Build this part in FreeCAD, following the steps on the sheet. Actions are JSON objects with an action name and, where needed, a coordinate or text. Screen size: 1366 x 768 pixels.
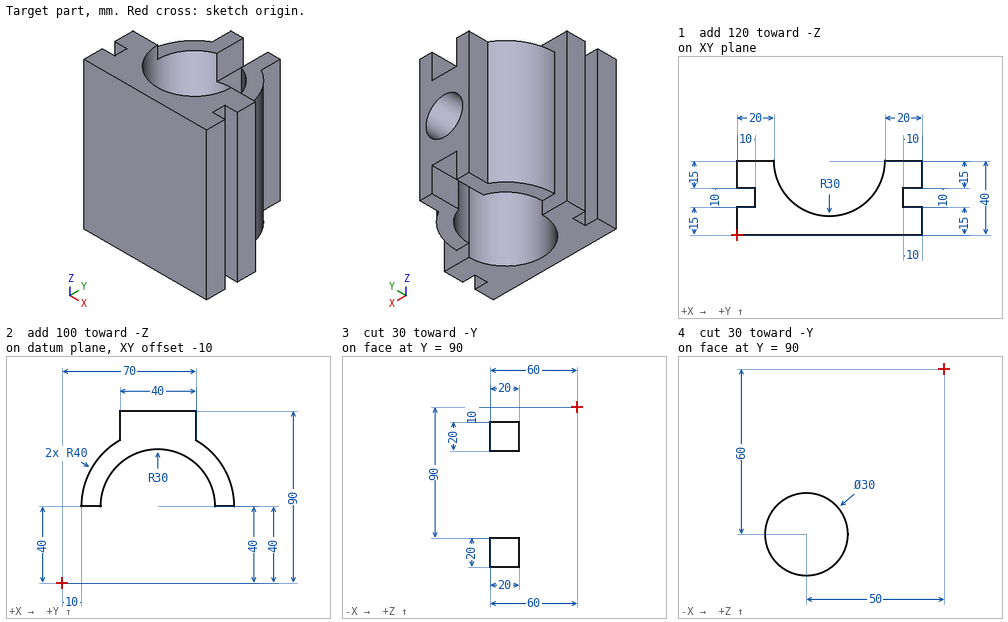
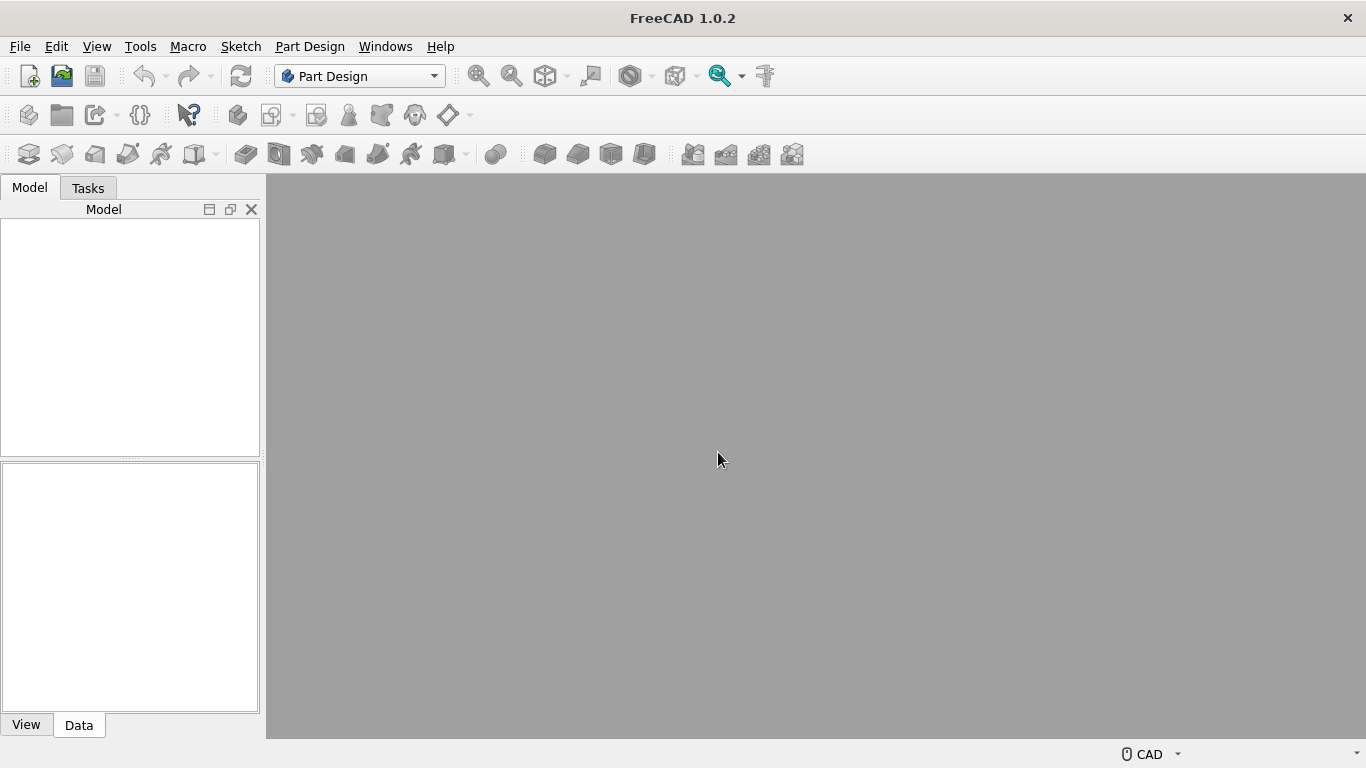
{"action": "left_click", "coordinate": [29, 76]}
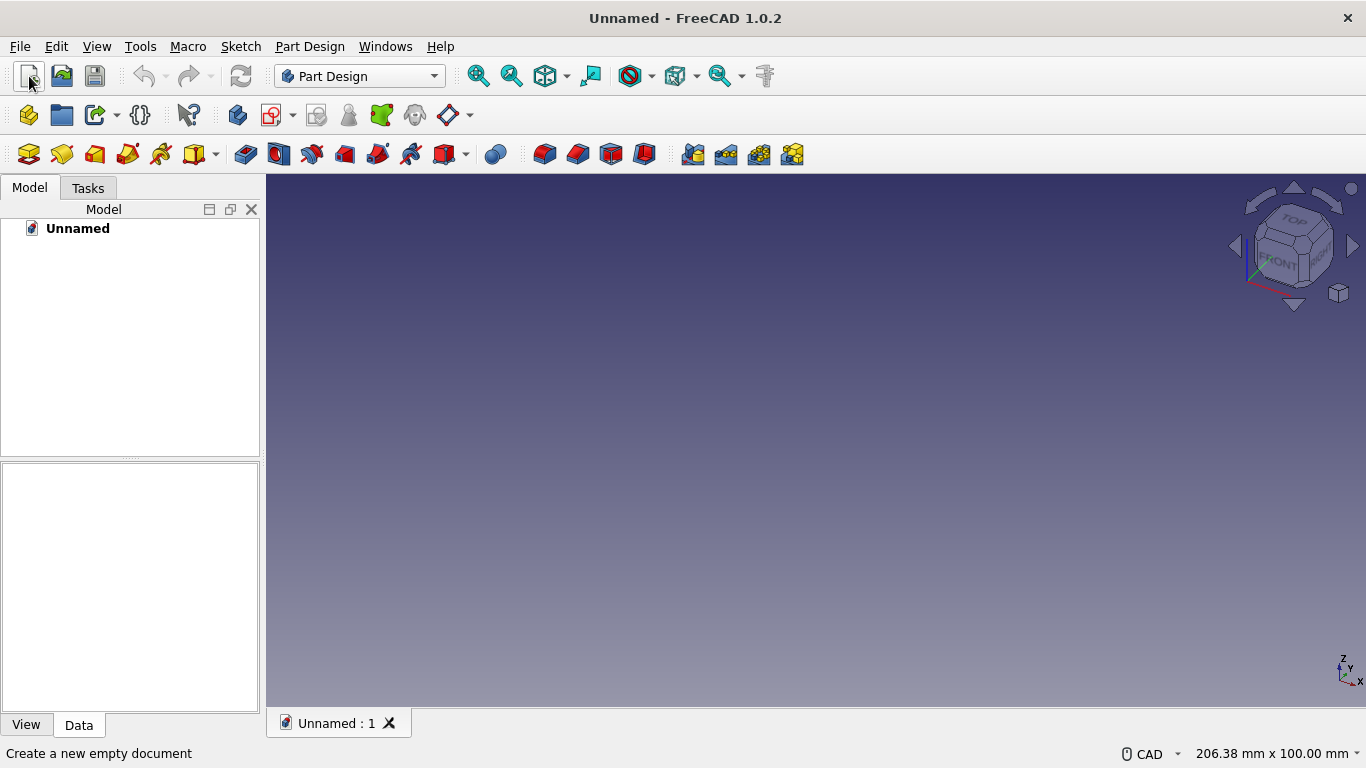
{"action": "left_click", "coordinate": [270, 116]}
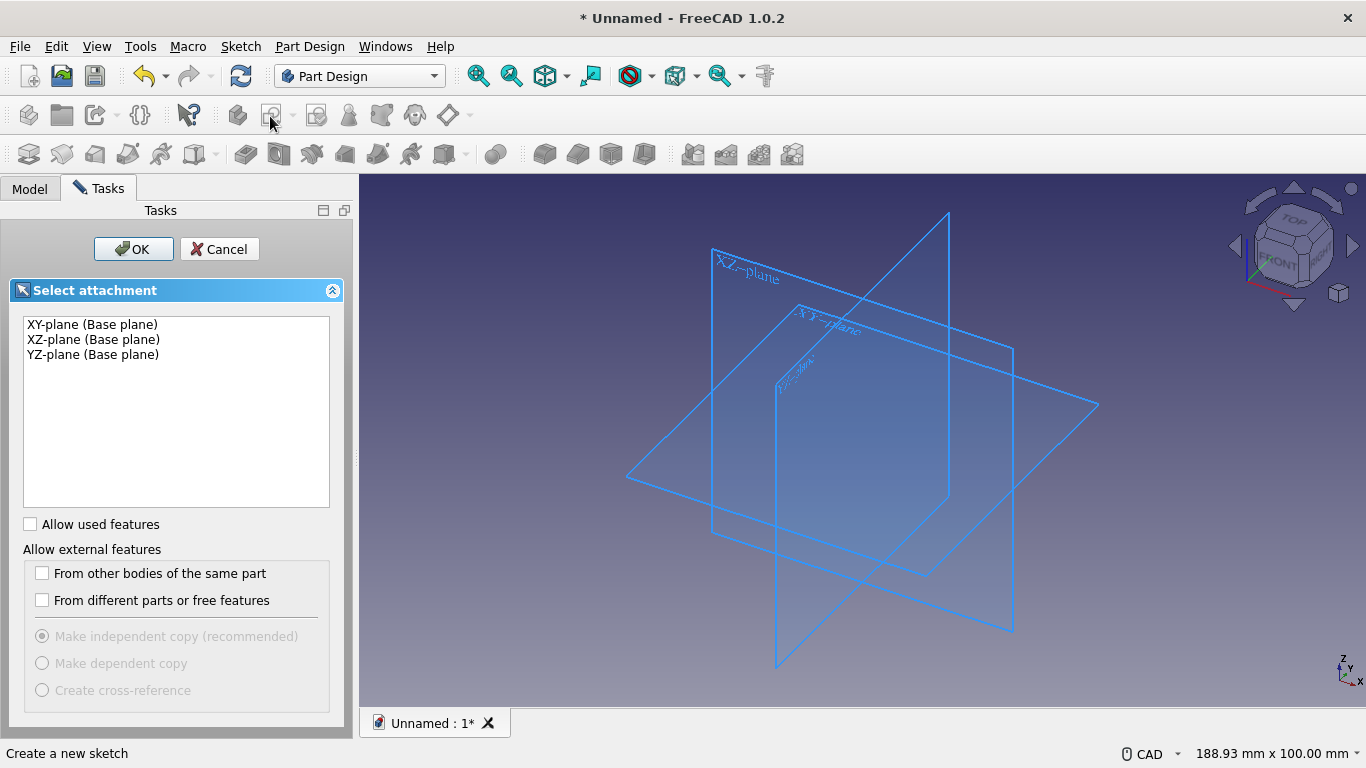
{"action": "left_click", "coordinate": [84, 324]}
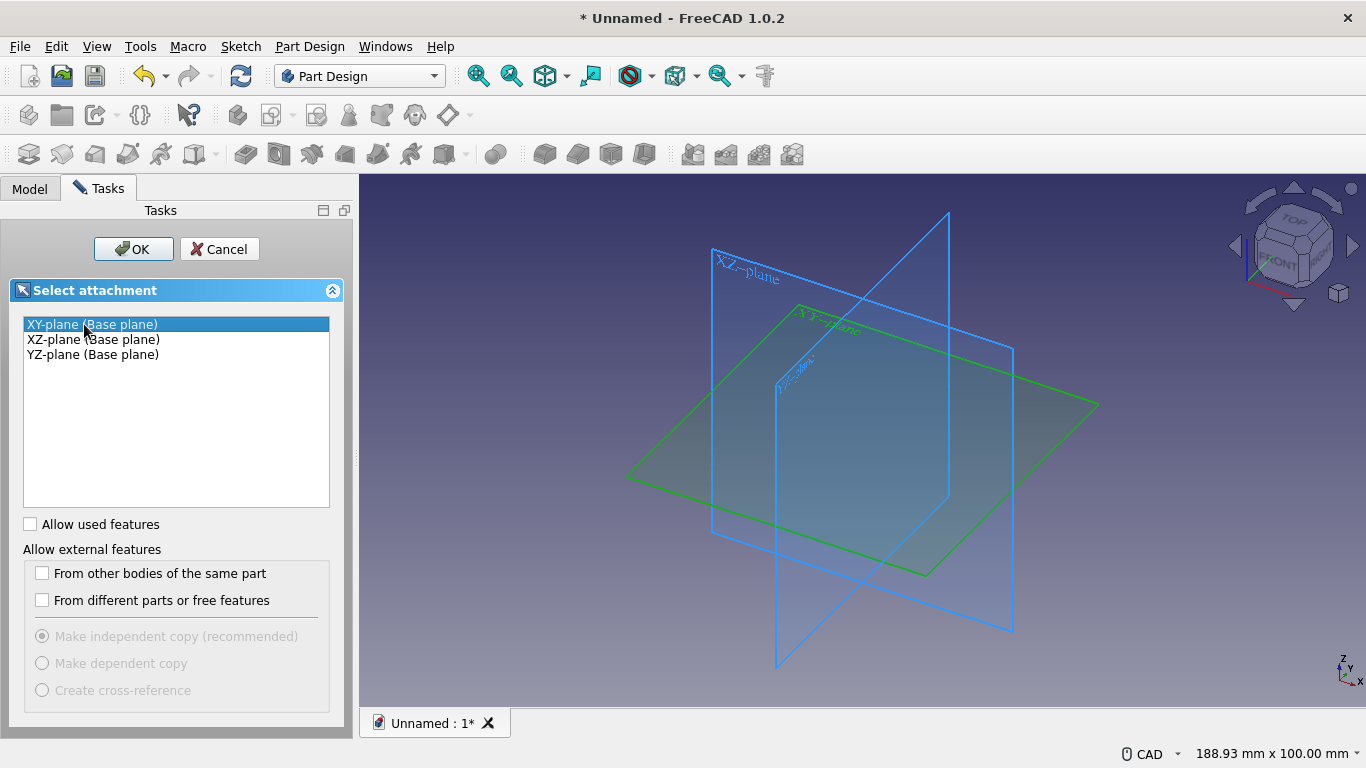
{"action": "left_click", "coordinate": [134, 249]}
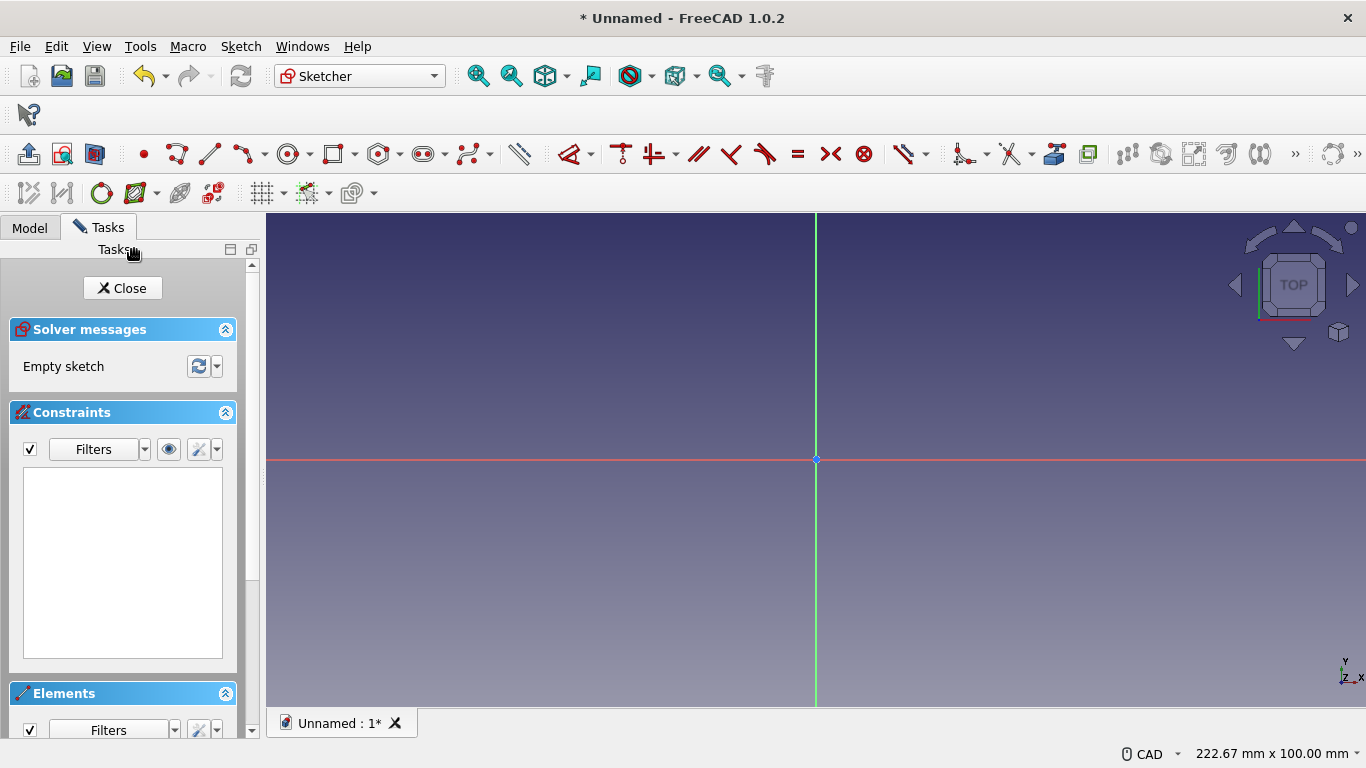
{"action": "scroll", "coordinate": [294, 679], "scroll_direction": "down", "scroll_amount": 1}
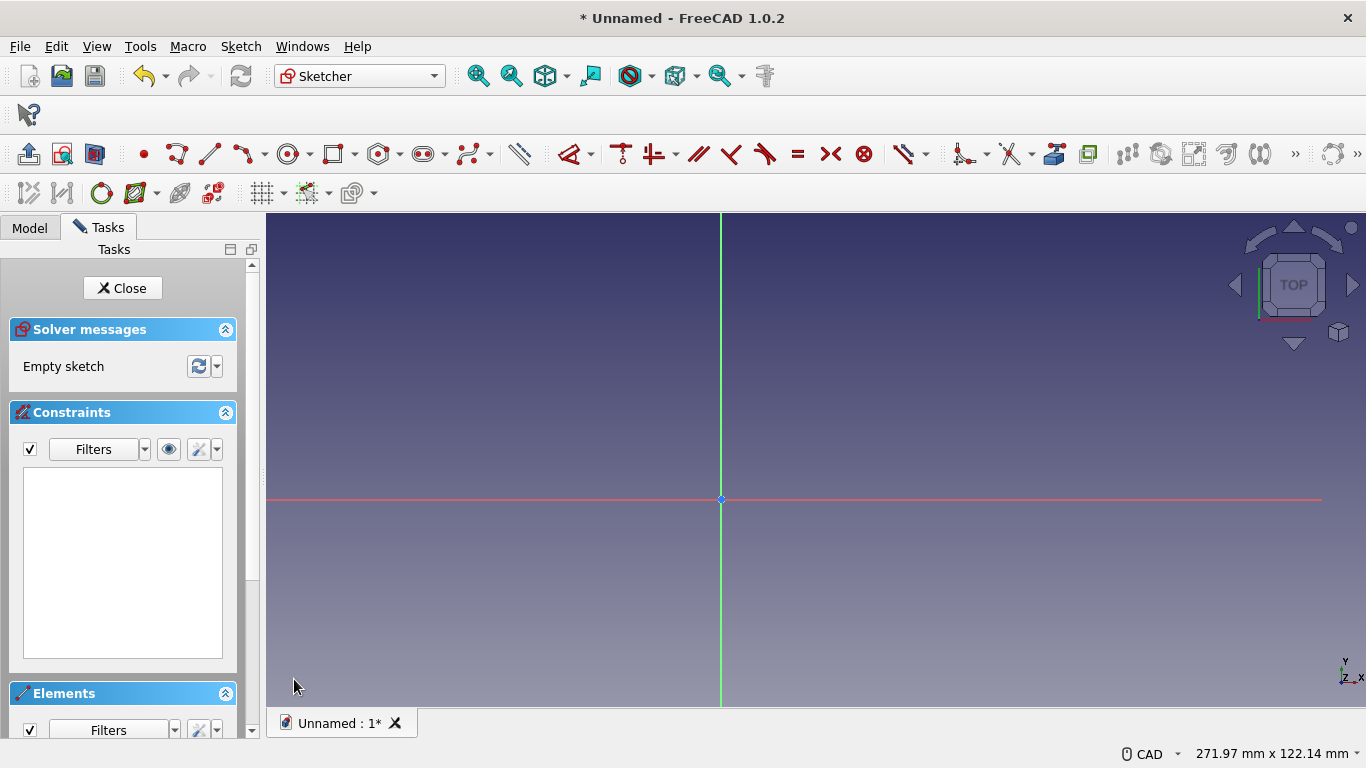
{"action": "scroll", "coordinate": [1201, 336], "scroll_direction": "up", "scroll_amount": 2}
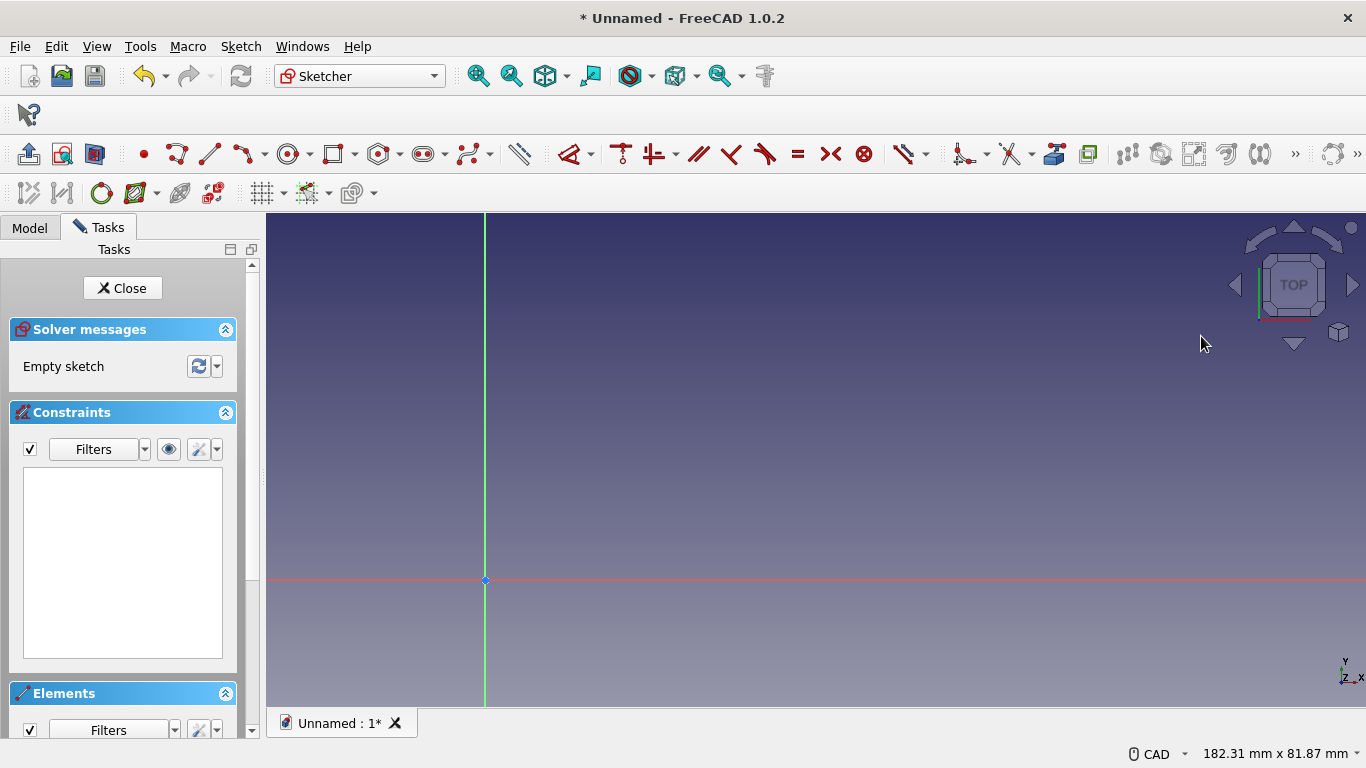
{"action": "left_click", "coordinate": [177, 154]}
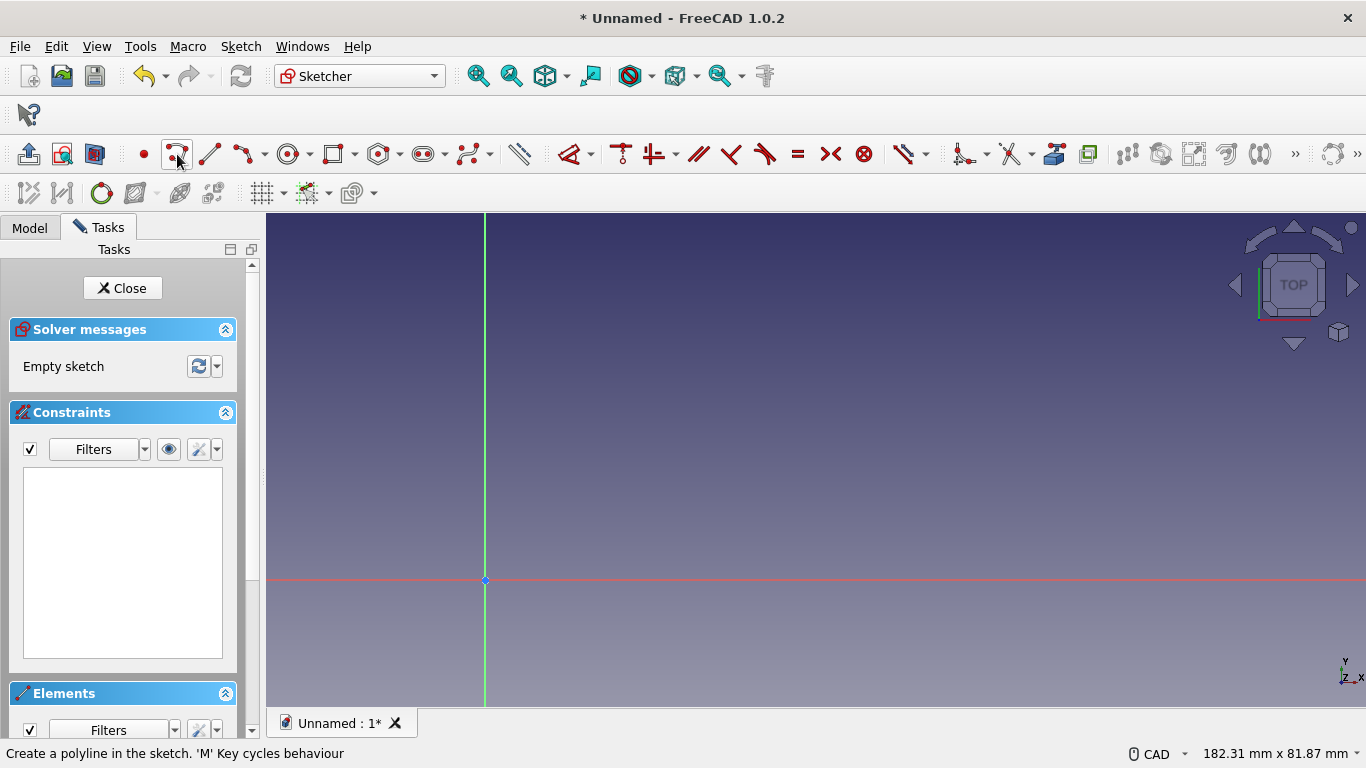
{"action": "left_click", "coordinate": [606, 339]}
{"action": "left_click", "coordinate": [485, 339]}
{"action": "left_click", "coordinate": [494, 429]}
{"action": "left_click", "coordinate": [545, 429]}
{"action": "left_click", "coordinate": [545, 490]}
{"action": "left_click", "coordinate": [485, 490]}
{"action": "left_click", "coordinate": [485, 580]}
{"action": "left_click", "coordinate": [1088, 571]}
{"action": "left_click", "coordinate": [1088, 490]}
{"action": "left_click", "coordinate": [1028, 490]}
{"action": "left_click", "coordinate": [1028, 429]}
{"action": "left_click", "coordinate": [1088, 429]}
{"action": "left_click", "coordinate": [1088, 339]}
{"action": "left_click", "coordinate": [968, 339]}
{"action": "right_click", "coordinate": [968, 339]}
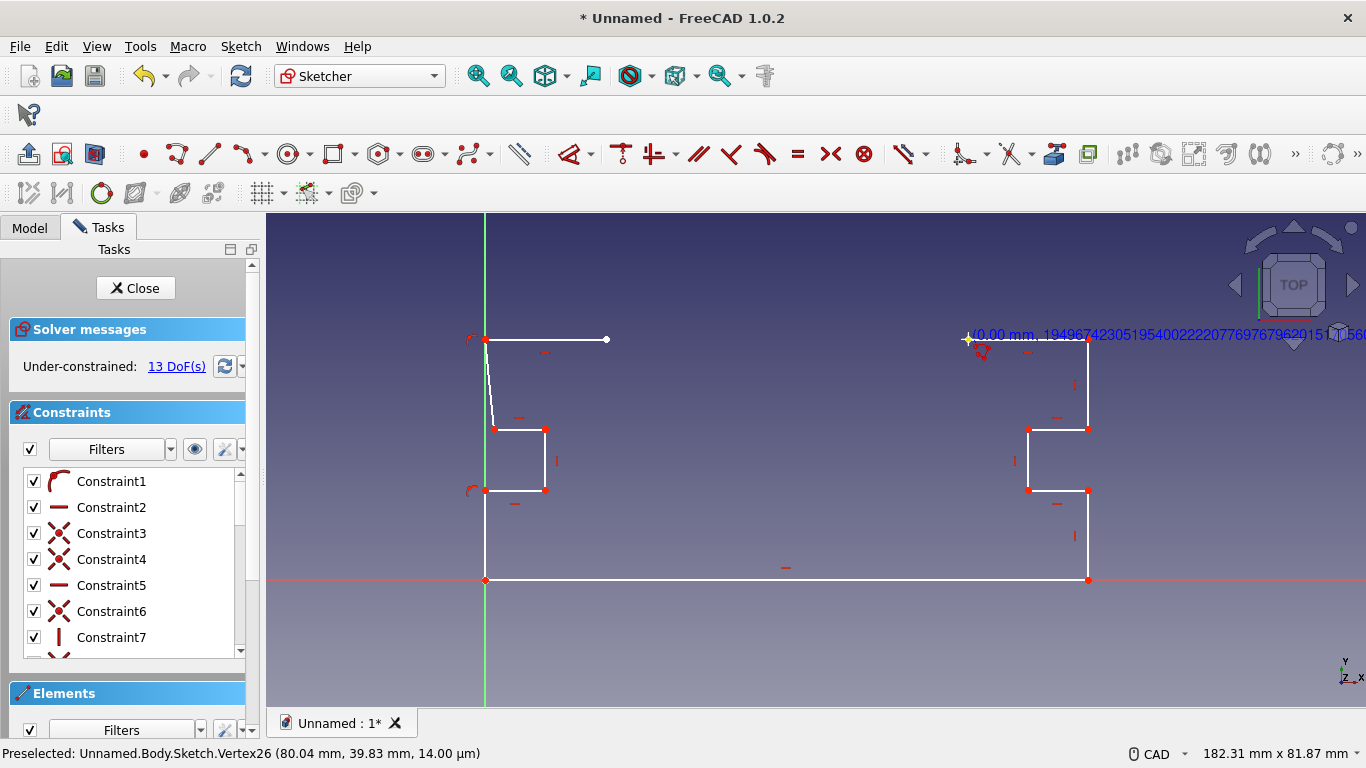
{"action": "left_click", "coordinate": [242, 154]}